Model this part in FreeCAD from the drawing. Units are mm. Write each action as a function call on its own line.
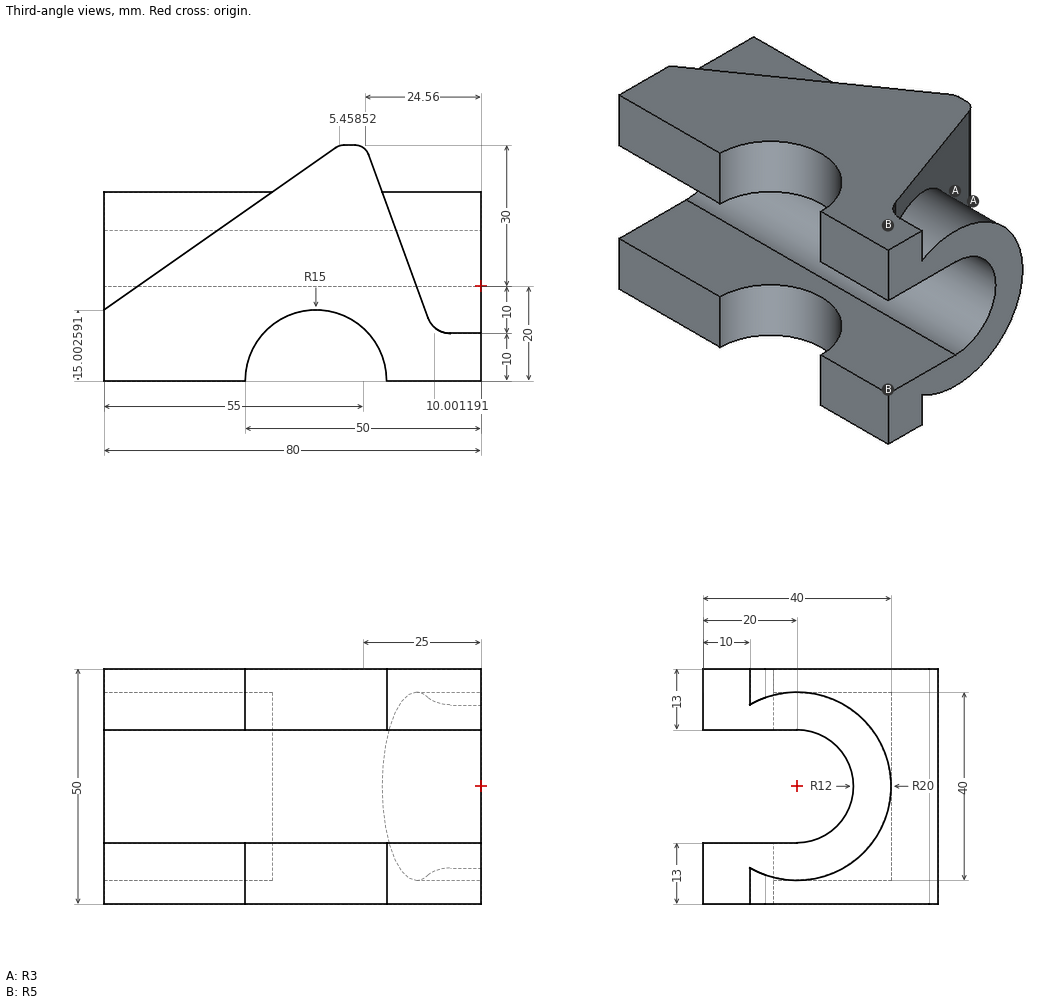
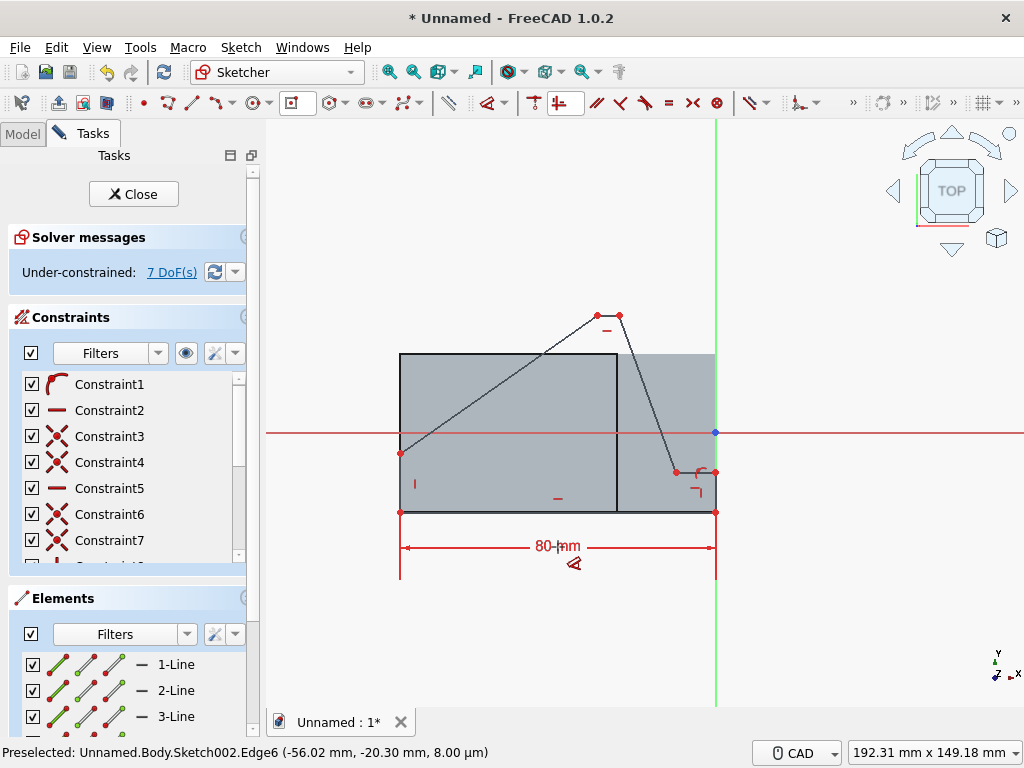
click(716, 501)
click(750, 493)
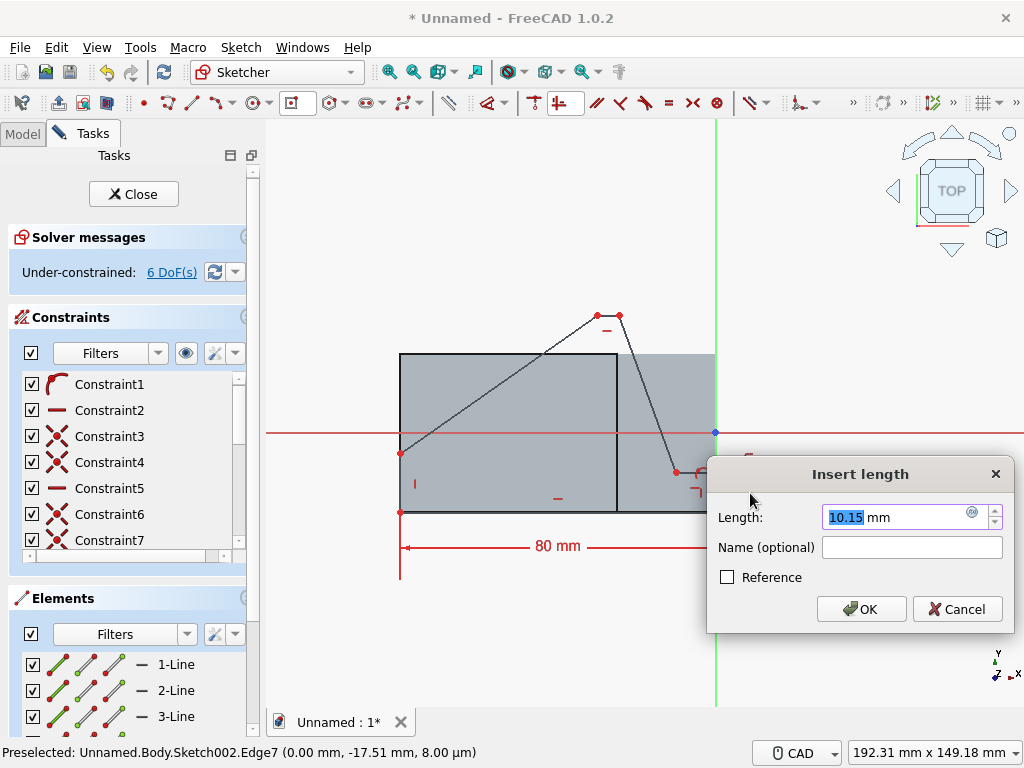
text(10)
key(Return)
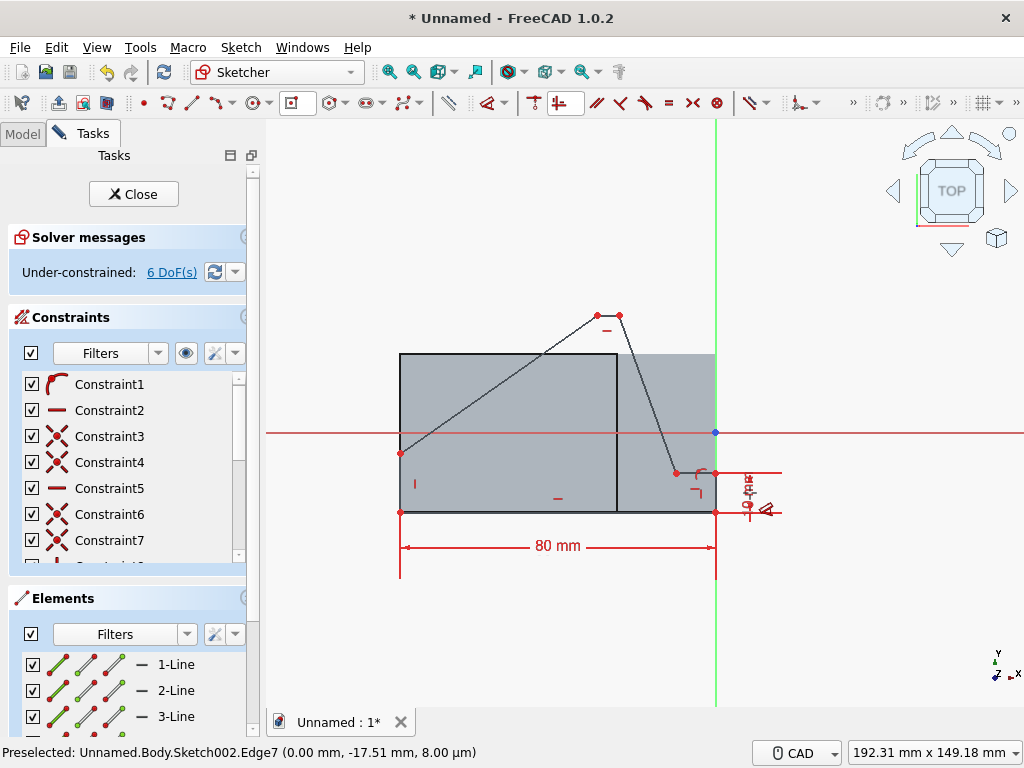
click(716, 473)
click(750, 453)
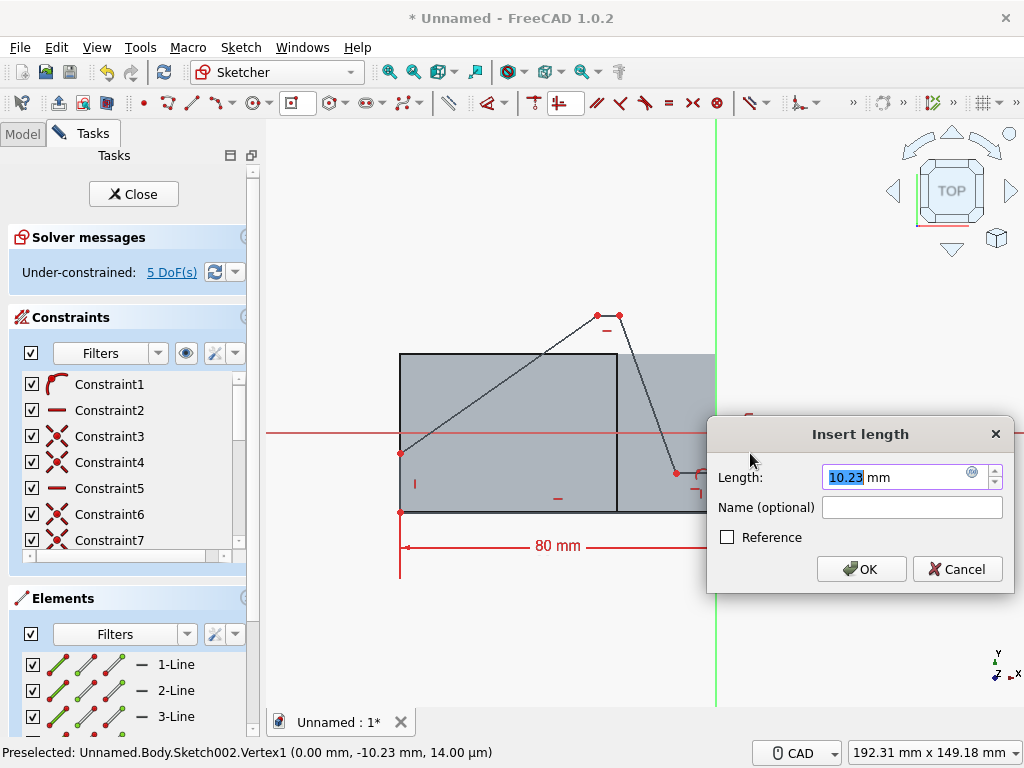
text(10)
key(Return)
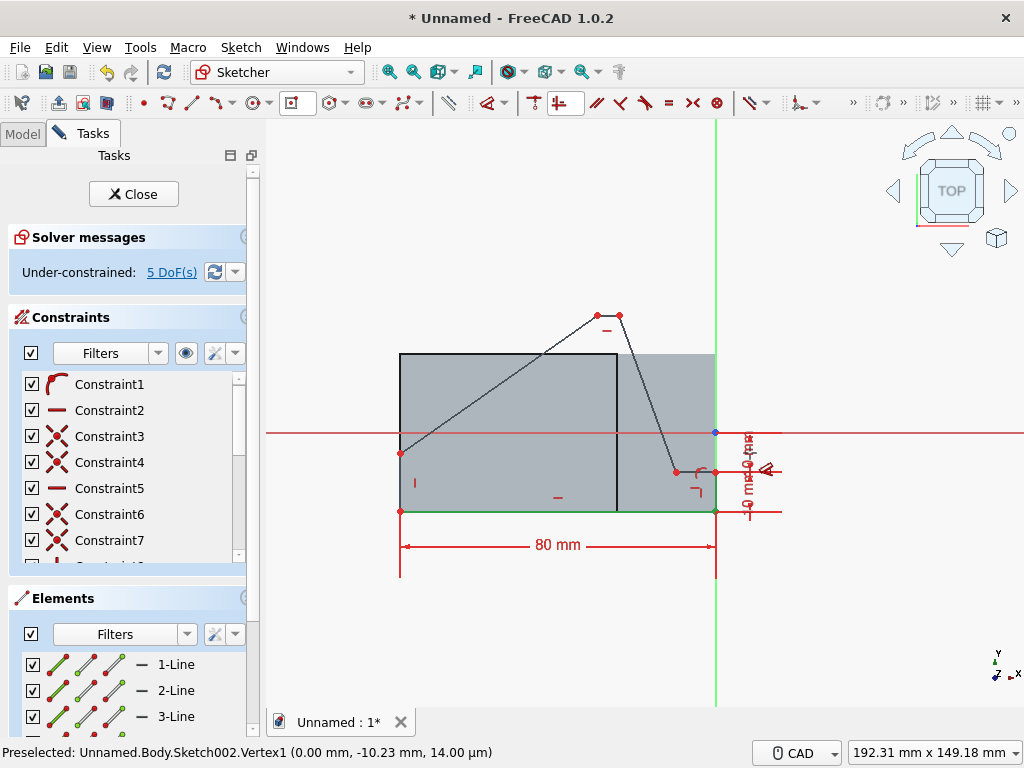
click(619, 316)
click(750, 374)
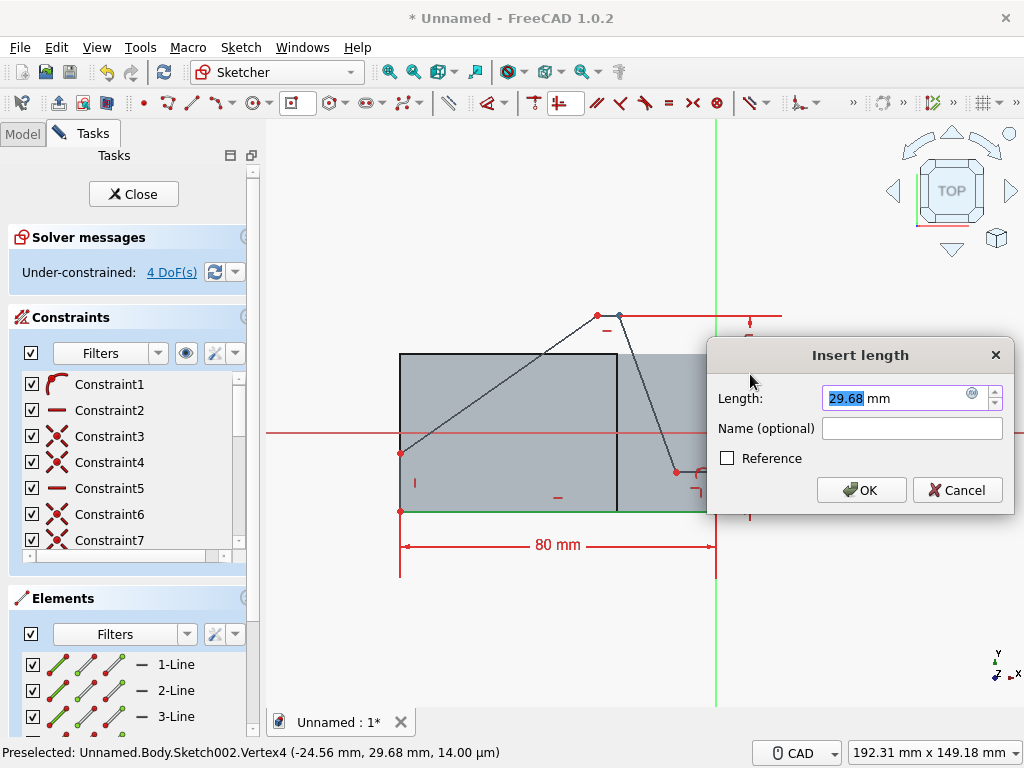
text(30)
key(Return)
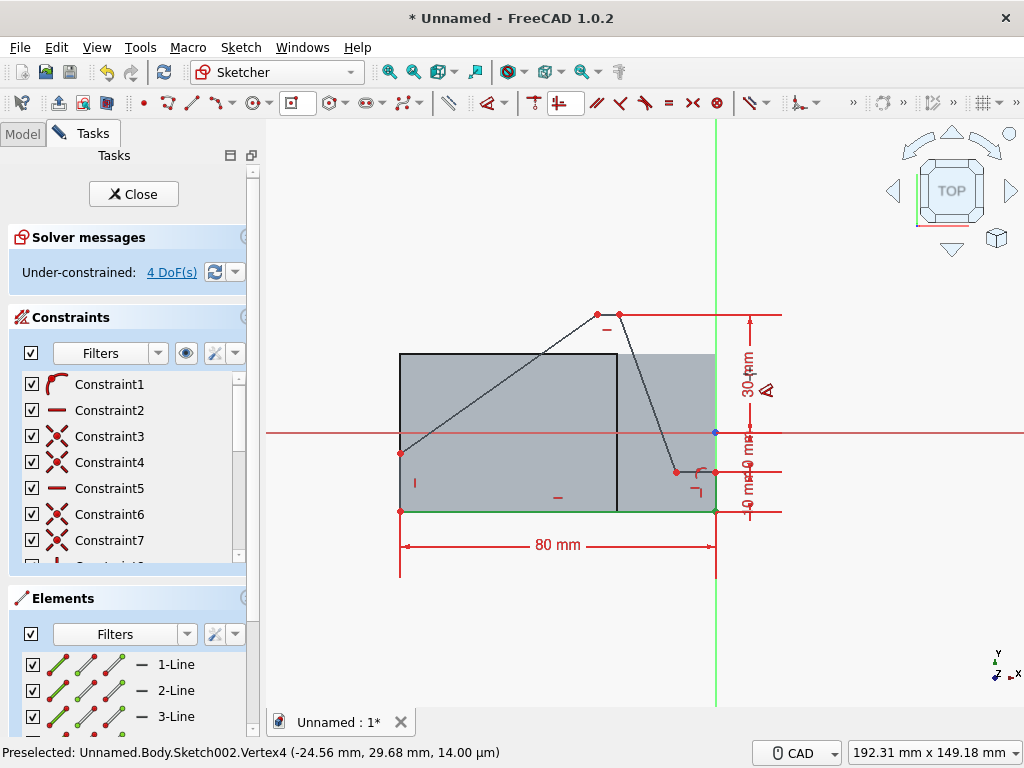
click(619, 315)
click(667, 281)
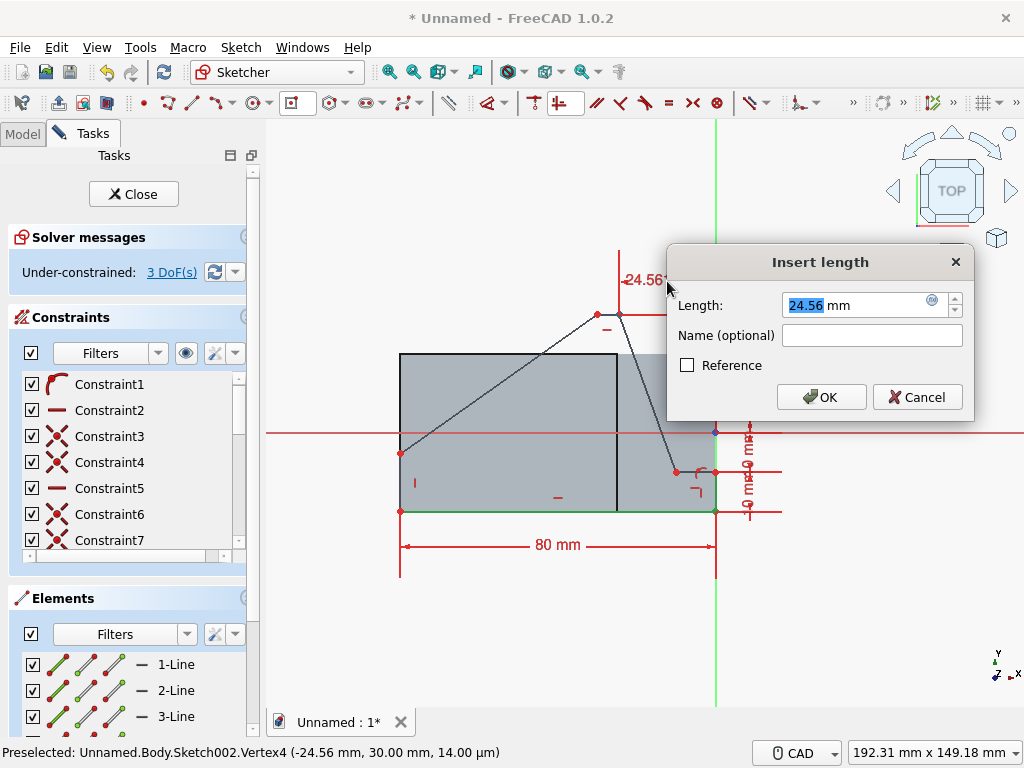
text(24.56)
key(Return)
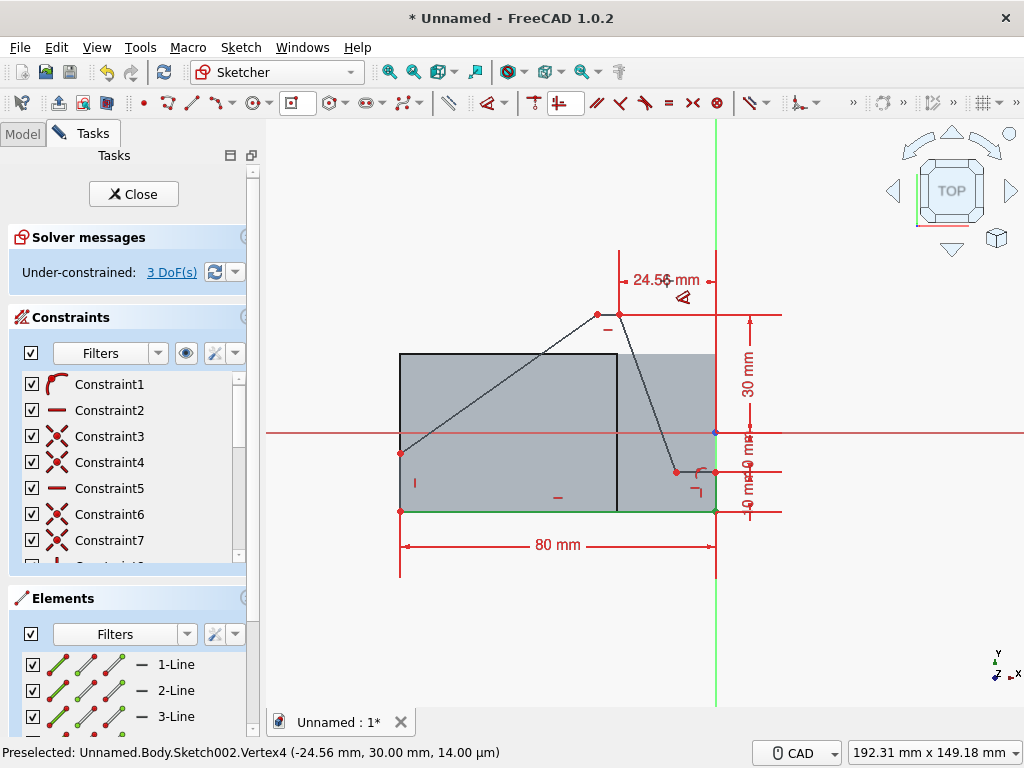
scroll(608, 315, up, 4)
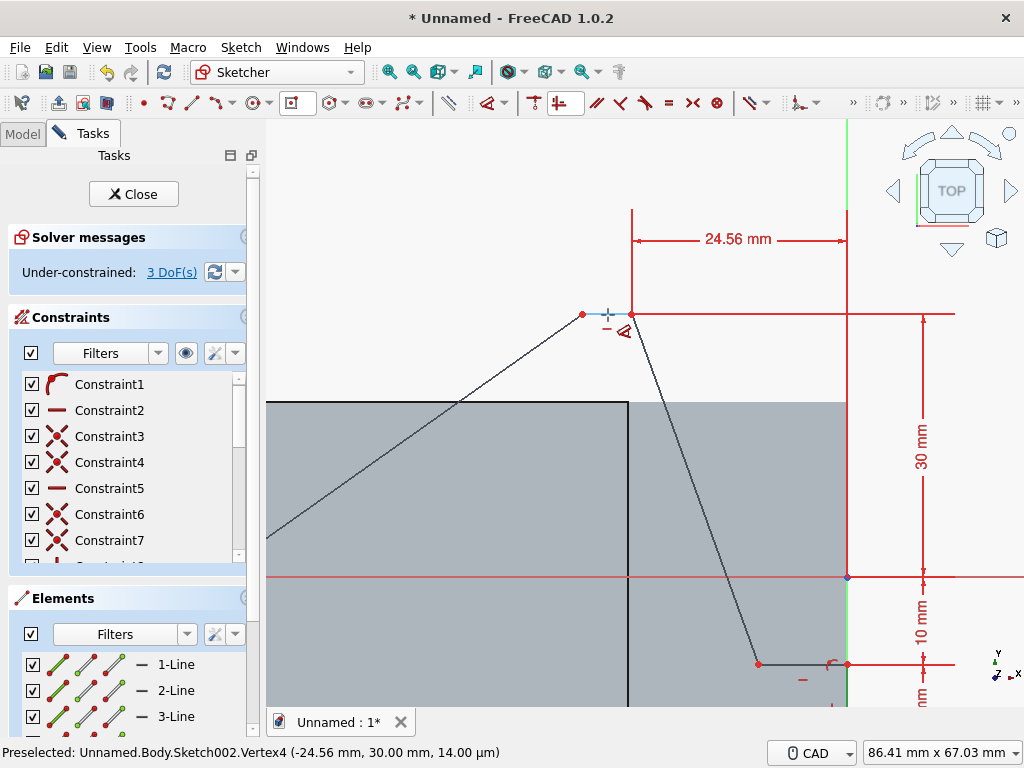
click(607, 314)
click(607, 280)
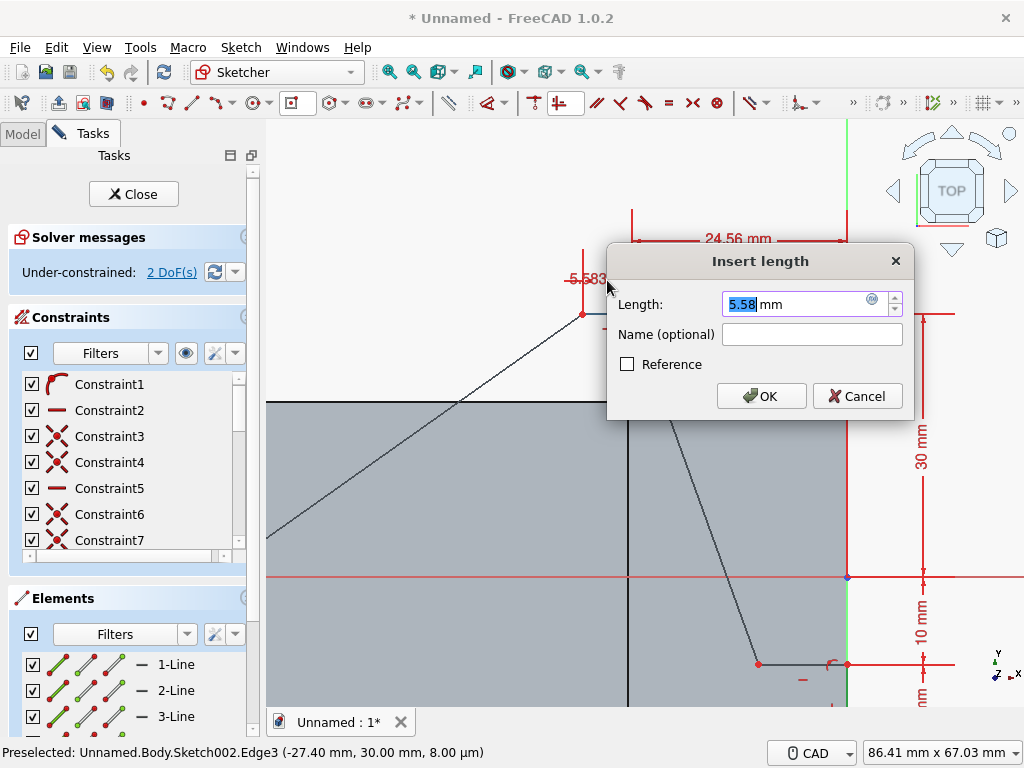
text(5.45852)
key(Return)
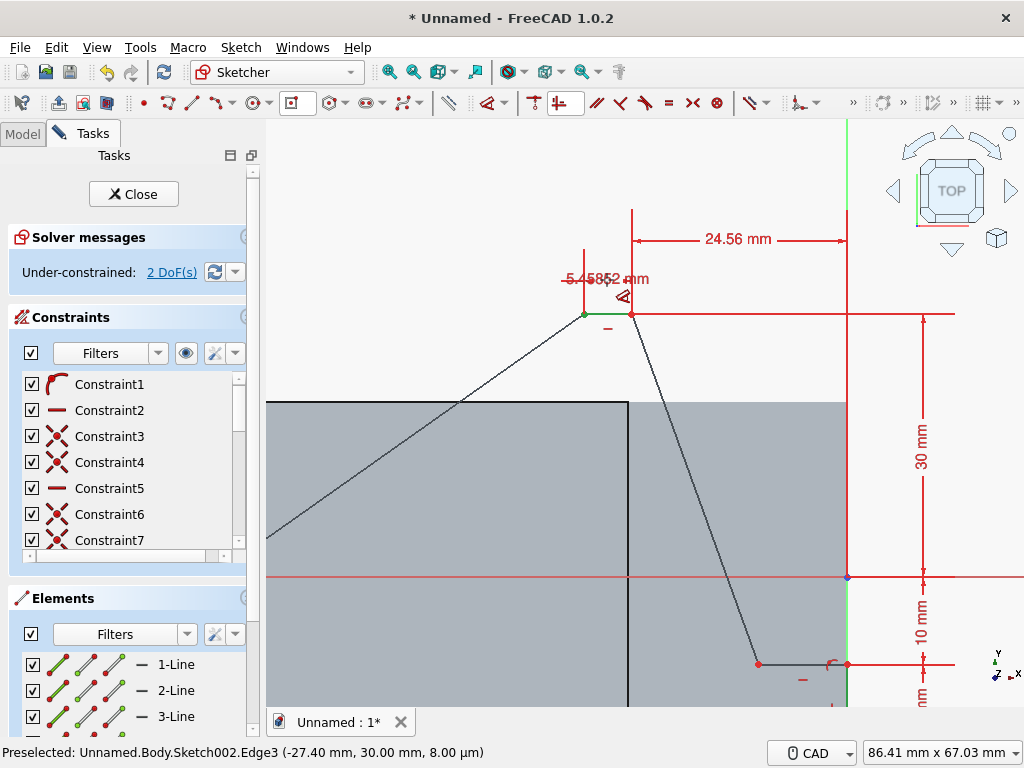
click(821, 665)
click(803, 631)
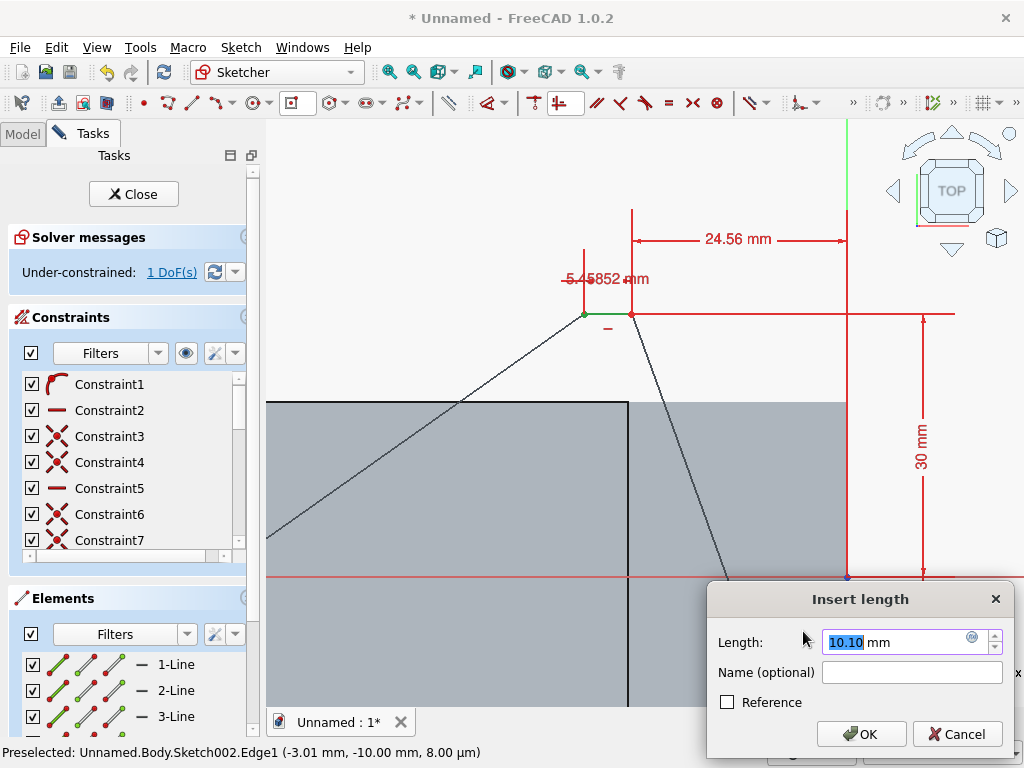
text(10.001191)
key(Return)